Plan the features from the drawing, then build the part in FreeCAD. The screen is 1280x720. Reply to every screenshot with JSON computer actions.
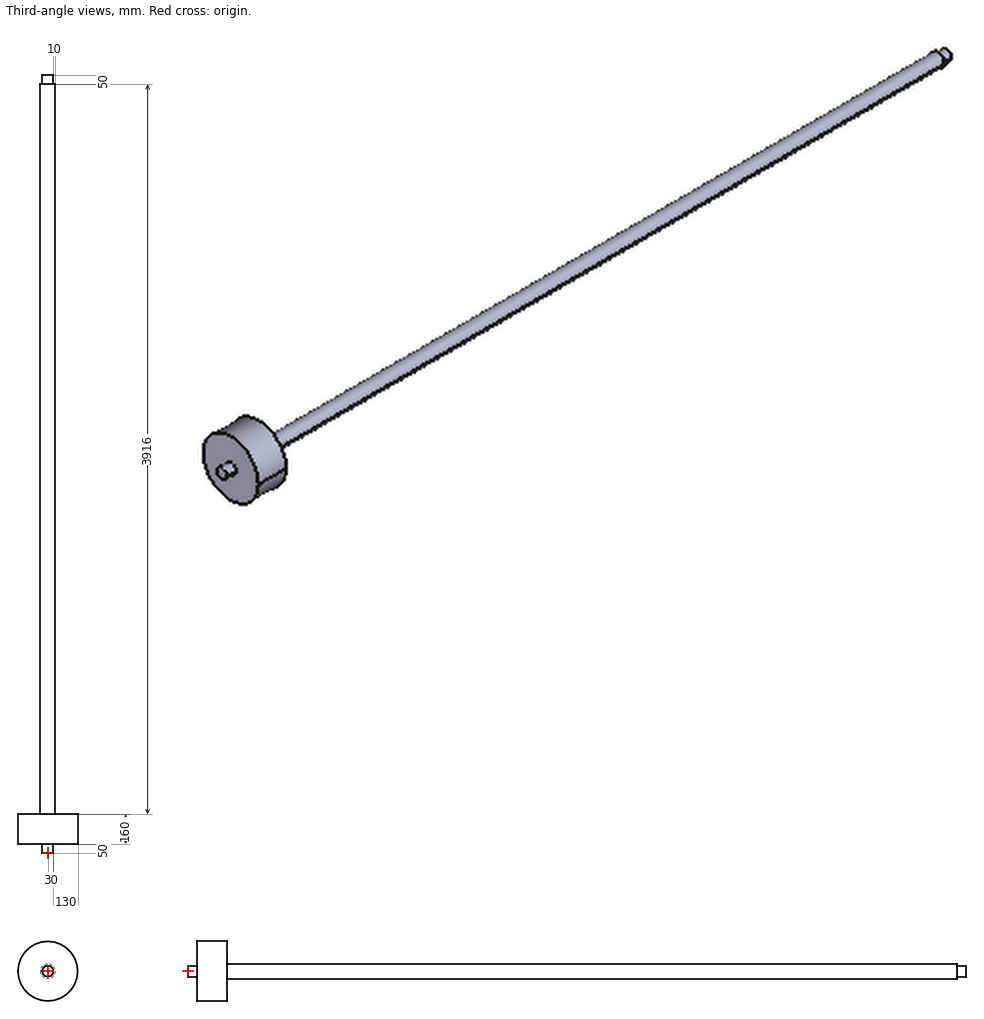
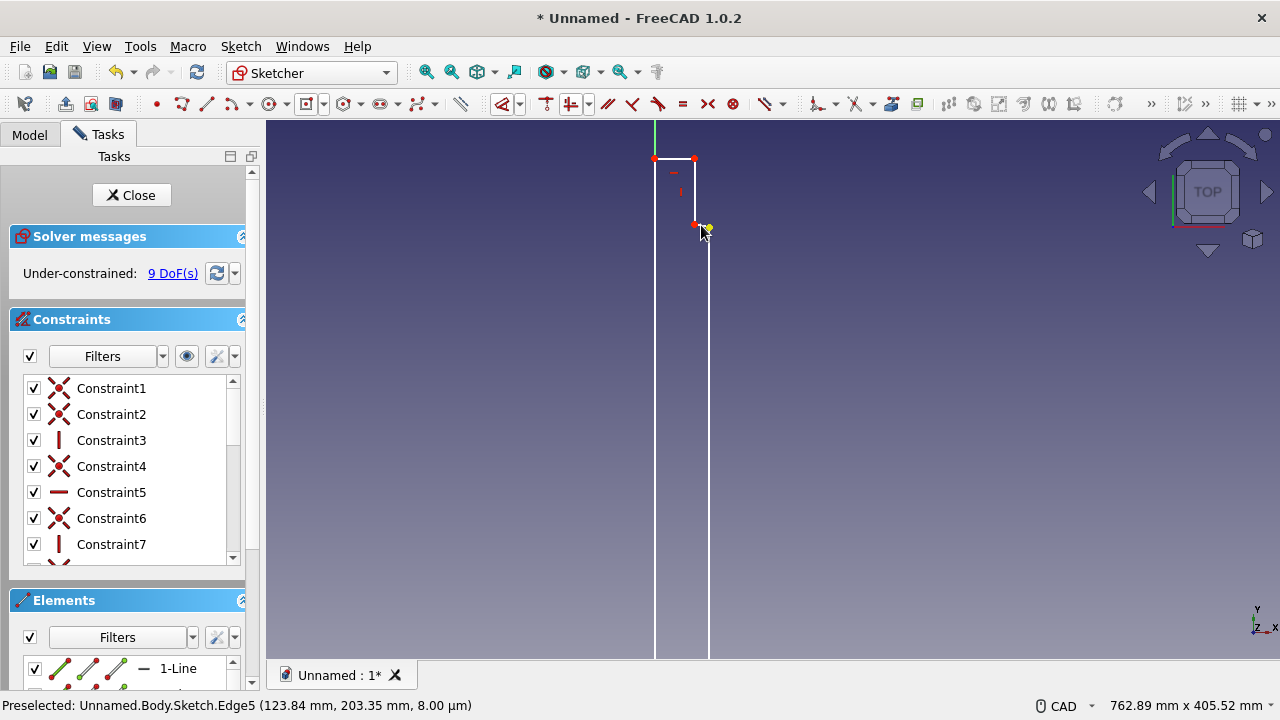
{"action": "left_click", "coordinate": [702, 226]}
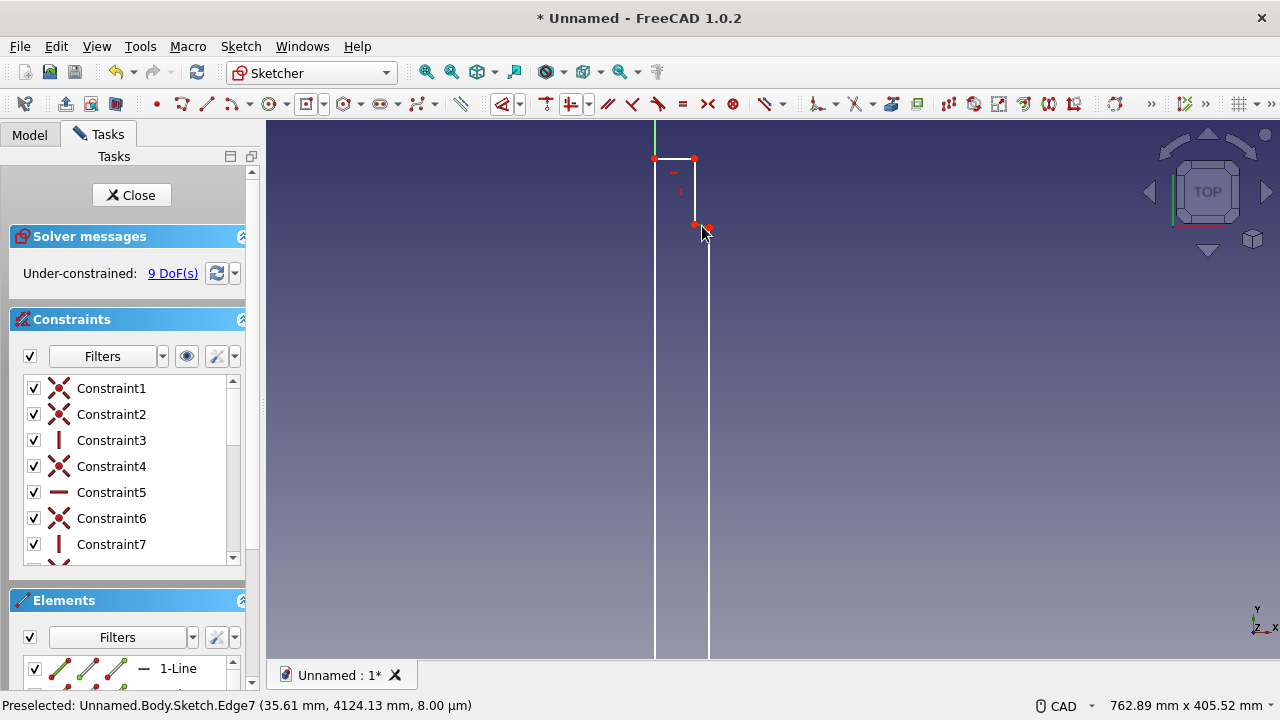
{"action": "key", "text": "h"}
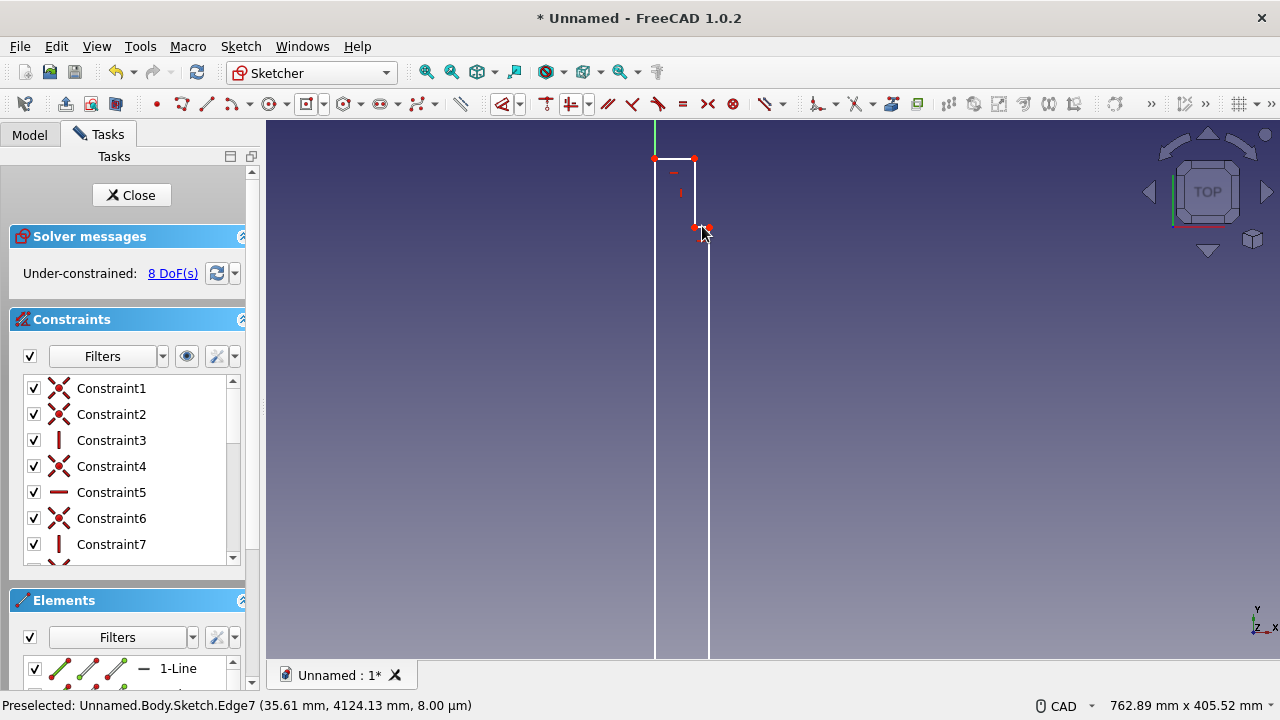
{"action": "left_click", "coordinate": [502, 104]}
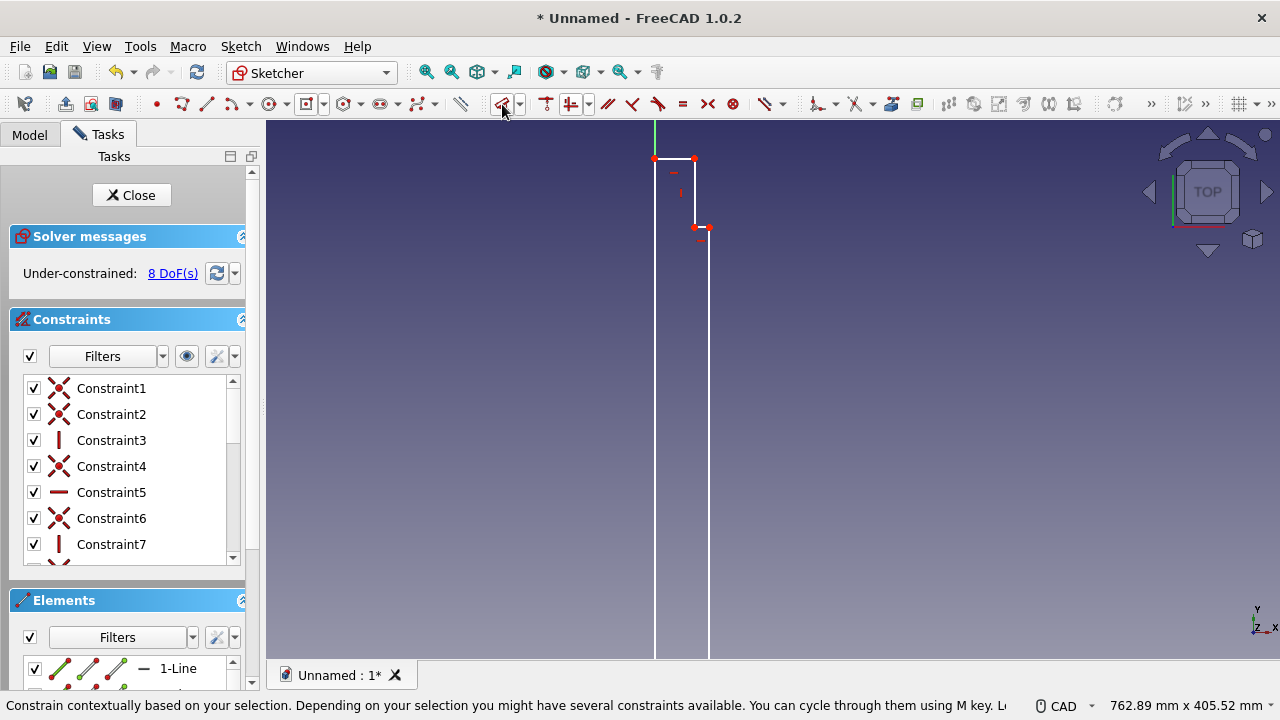
{"action": "scroll", "coordinate": [701, 225], "scroll_direction": "down", "scroll_amount": 14}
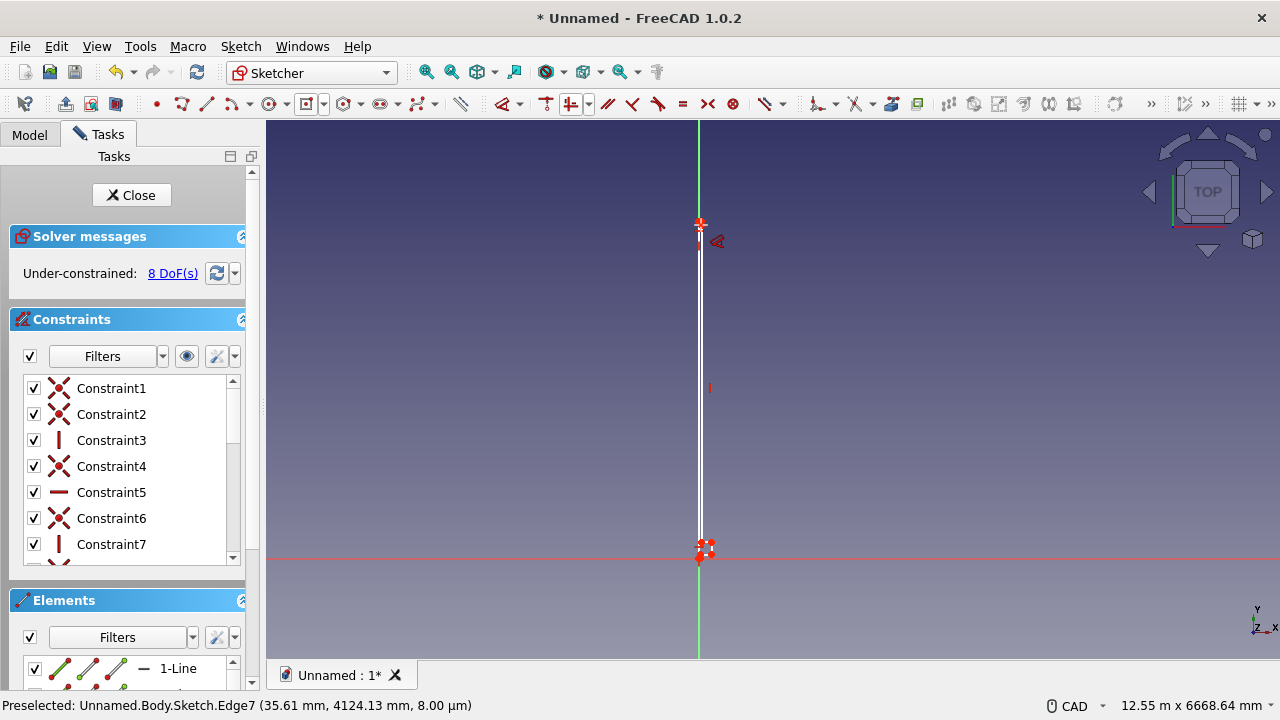
{"action": "scroll", "coordinate": [699, 559], "scroll_direction": "up", "scroll_amount": 14}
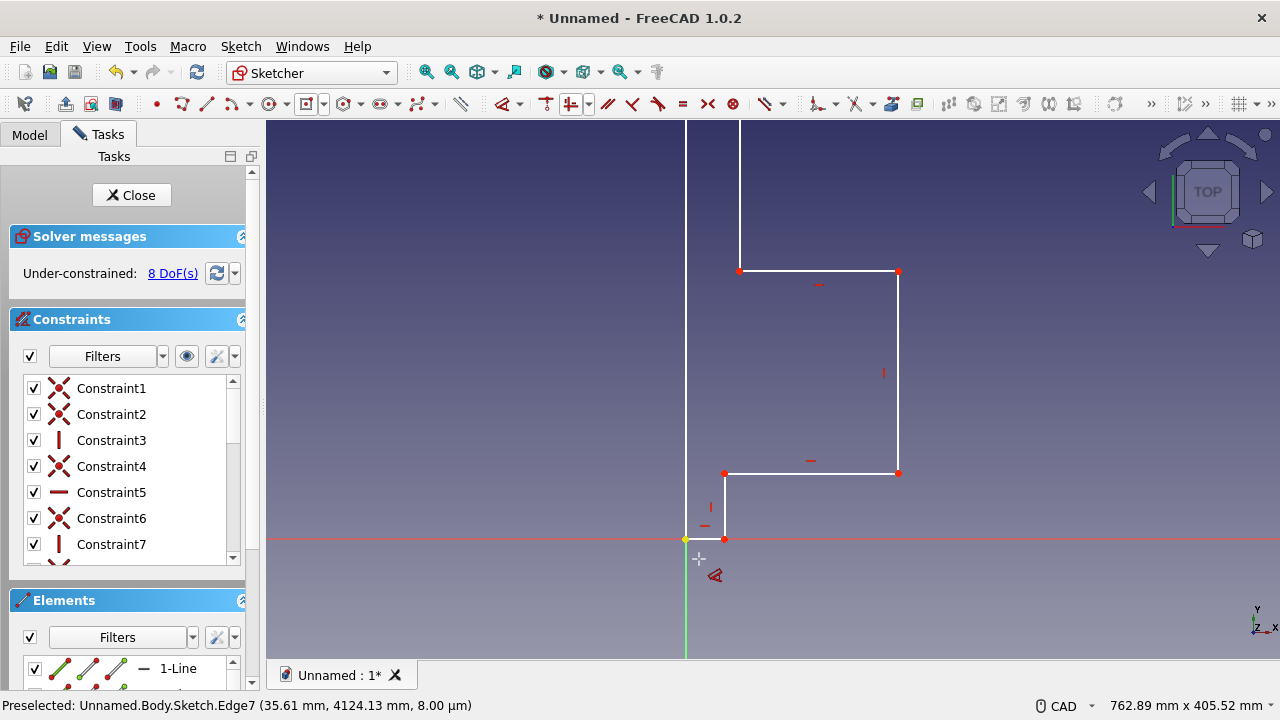
{"action": "left_click", "coordinate": [698, 539]}
{"action": "left_click", "coordinate": [705, 573]}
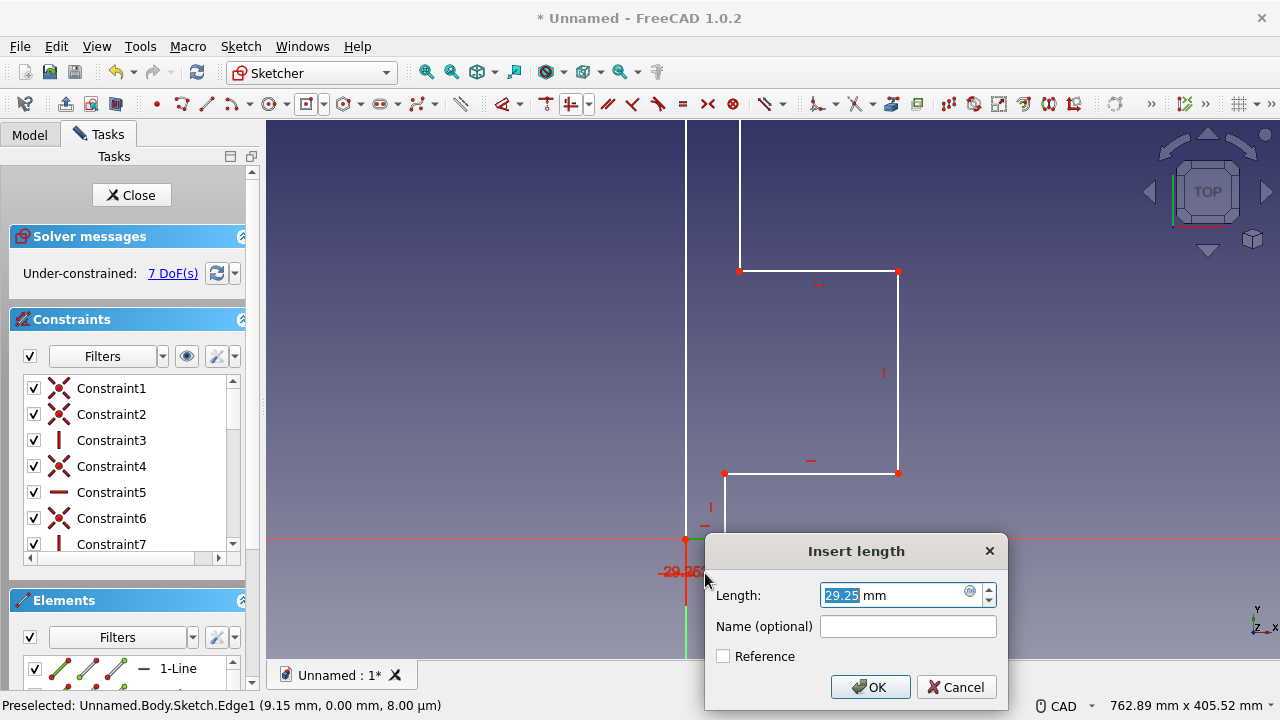
{"action": "type", "text": "30"}
{"action": "key", "text": "Return"}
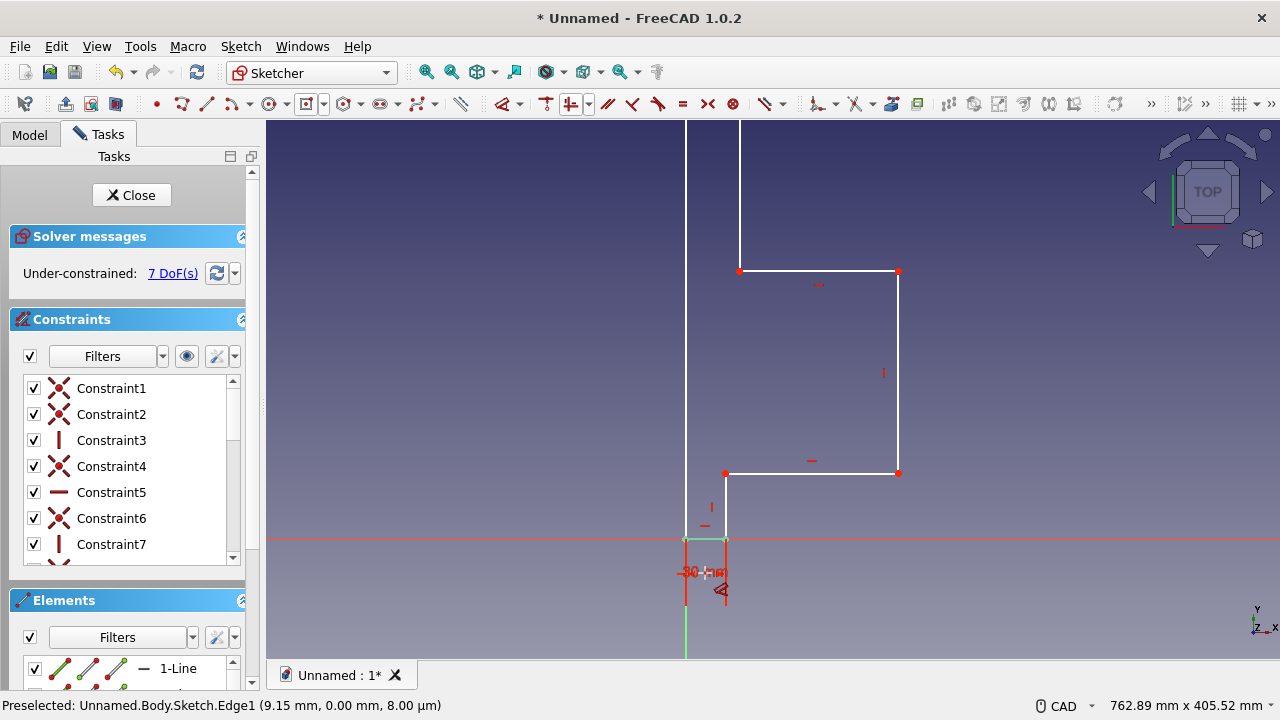
{"action": "left_click", "coordinate": [726, 520]}
{"action": "left_click", "coordinate": [760, 507]}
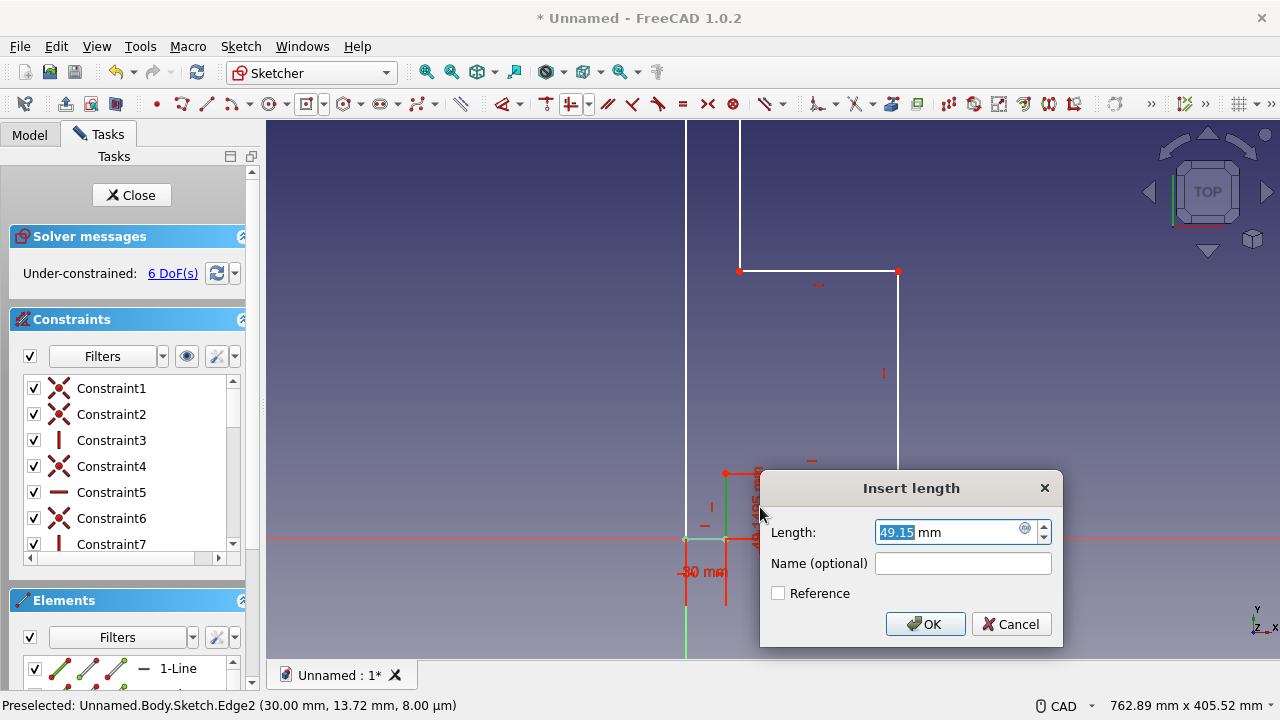
{"action": "type", "text": "50"}
{"action": "key", "text": "Return"}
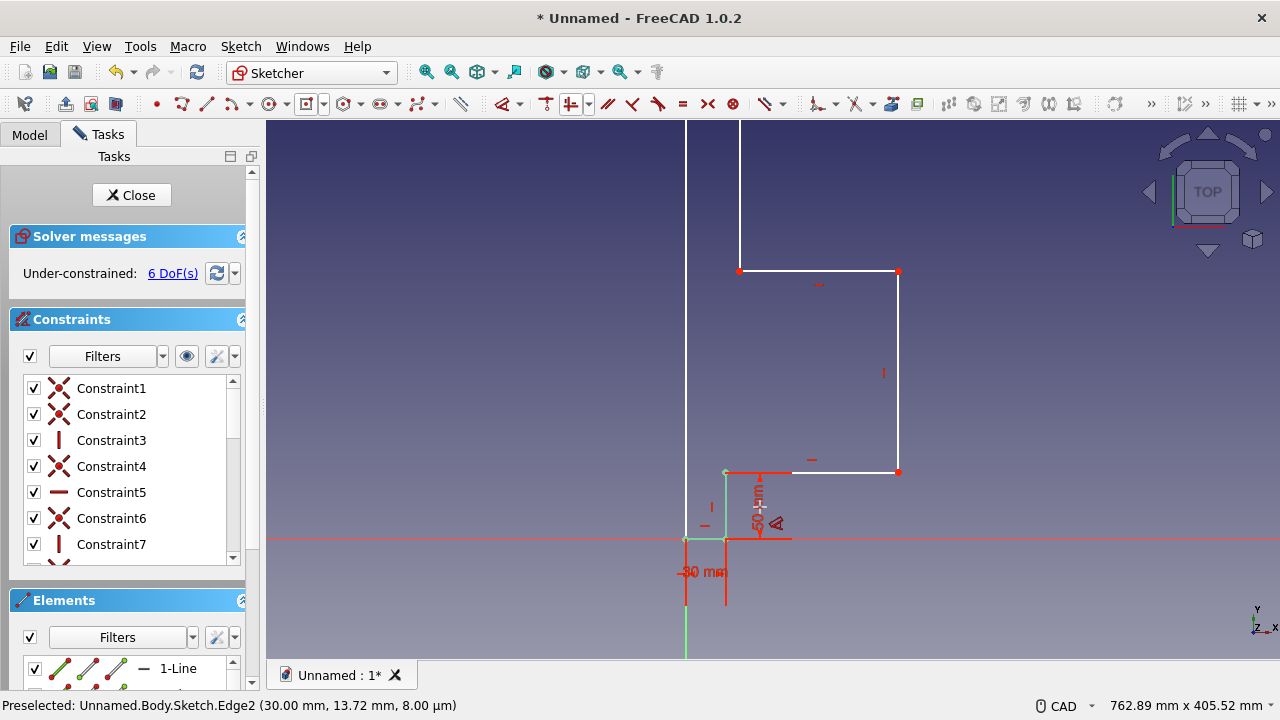
{"action": "scroll", "coordinate": [699, 559], "scroll_direction": "down", "scroll_amount": 14}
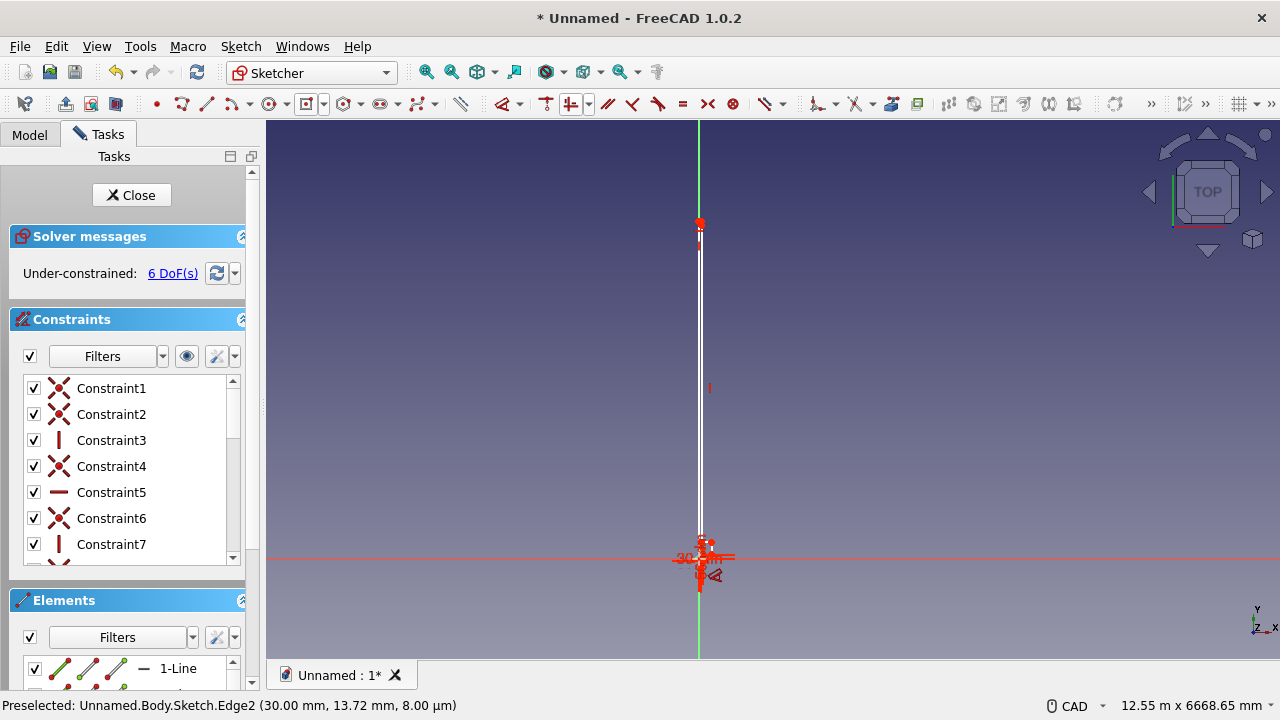
{"action": "scroll", "coordinate": [701, 225], "scroll_direction": "up", "scroll_amount": 20}